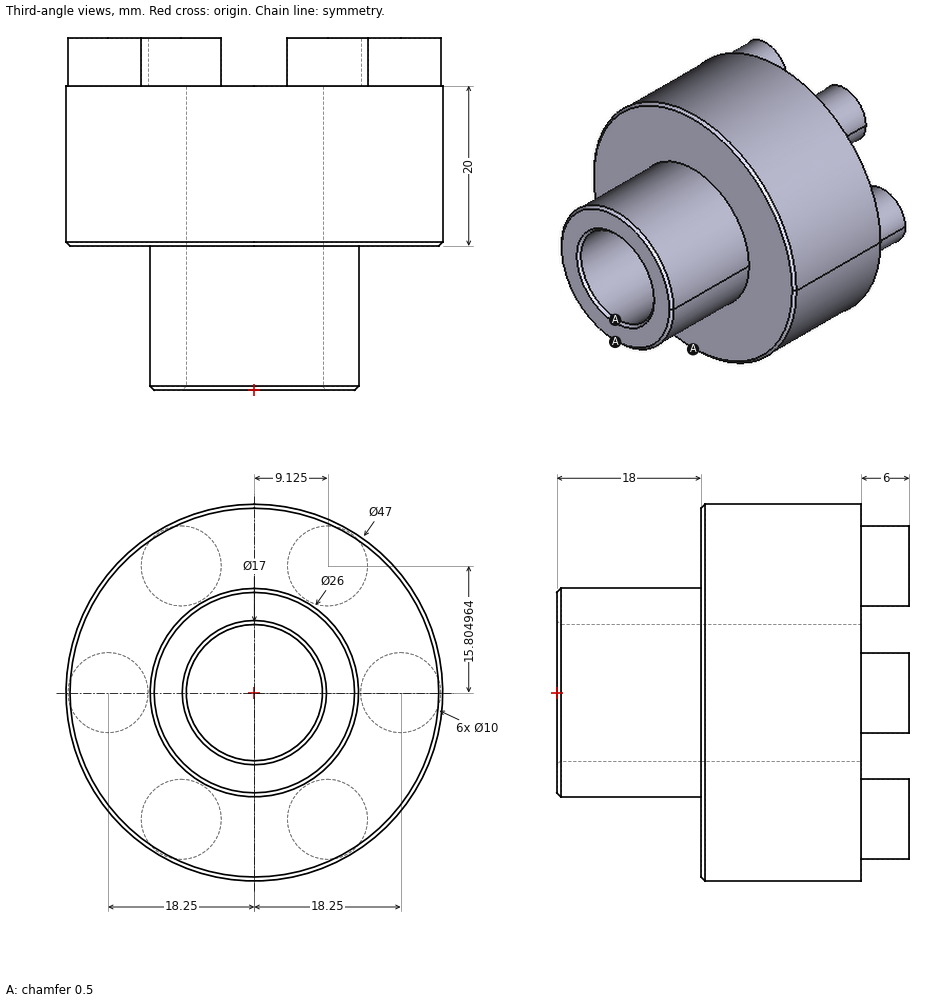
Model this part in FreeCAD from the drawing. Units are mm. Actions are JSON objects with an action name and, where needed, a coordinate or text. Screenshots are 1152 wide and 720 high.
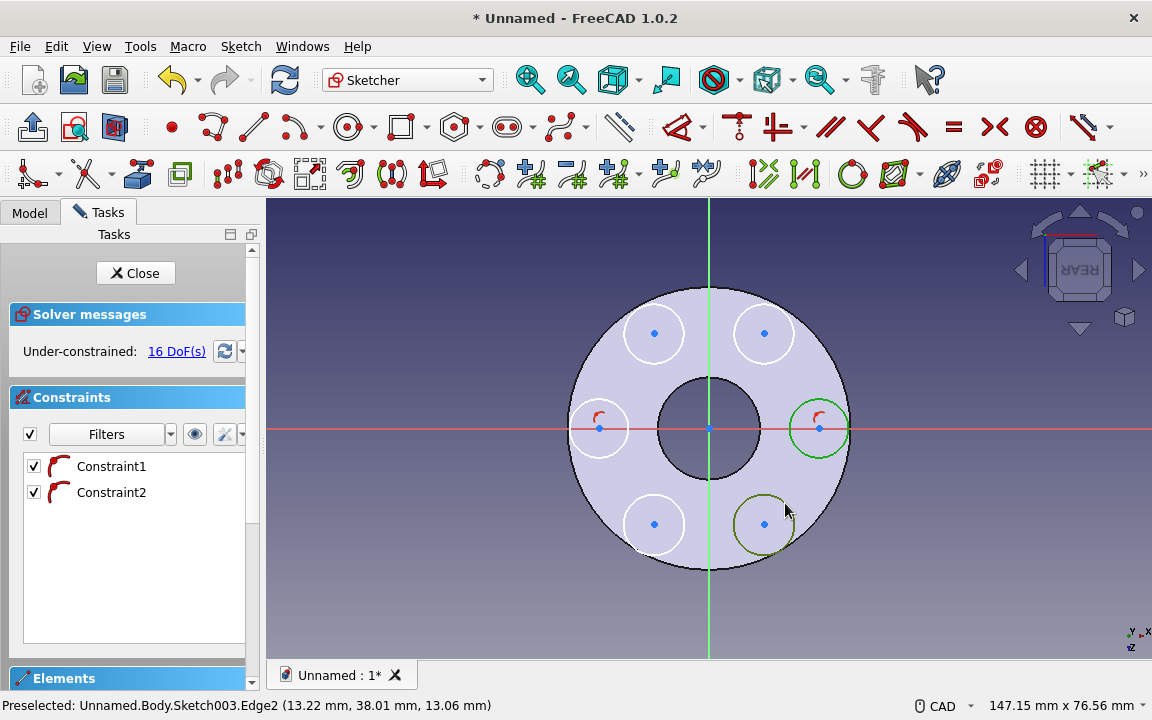
{"action": "left_click", "coordinate": [675, 503]}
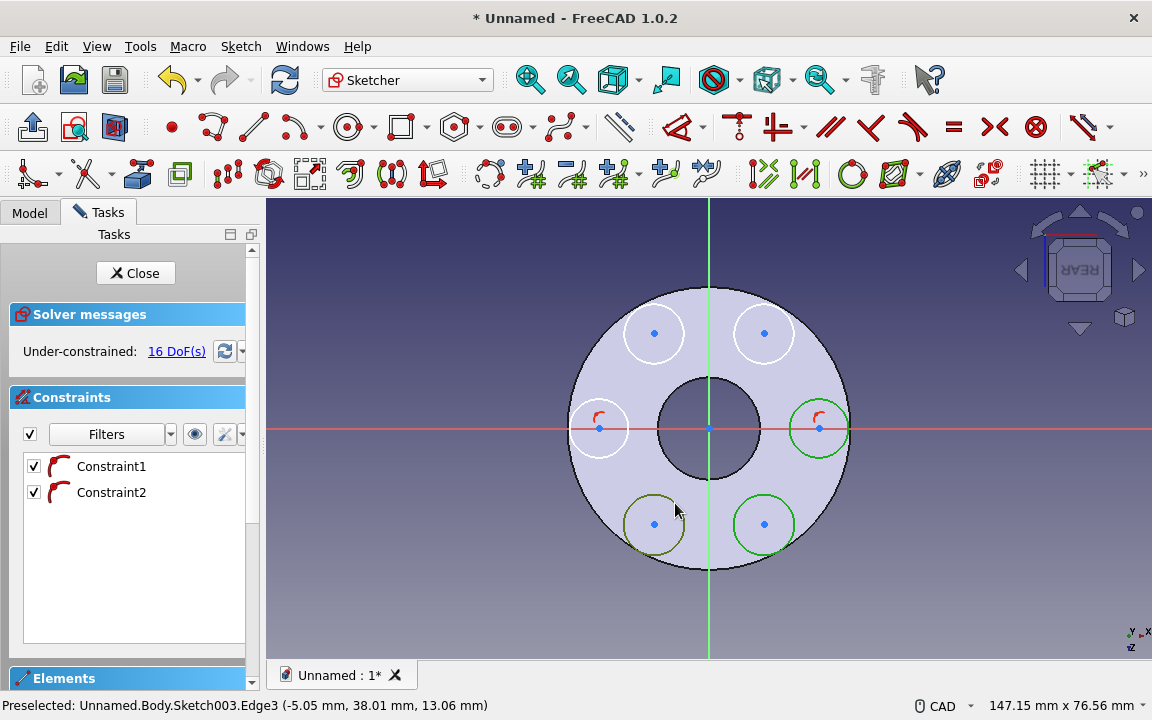
{"action": "left_click", "coordinate": [620, 408]}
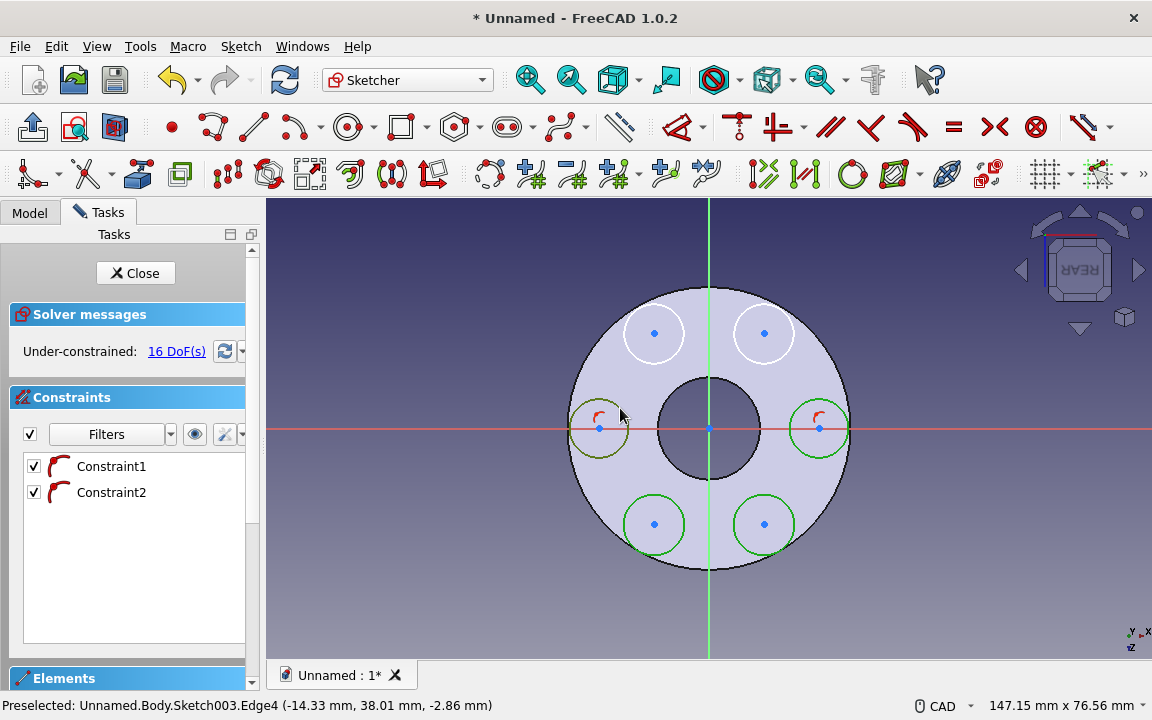
{"action": "left_click", "coordinate": [675, 313]}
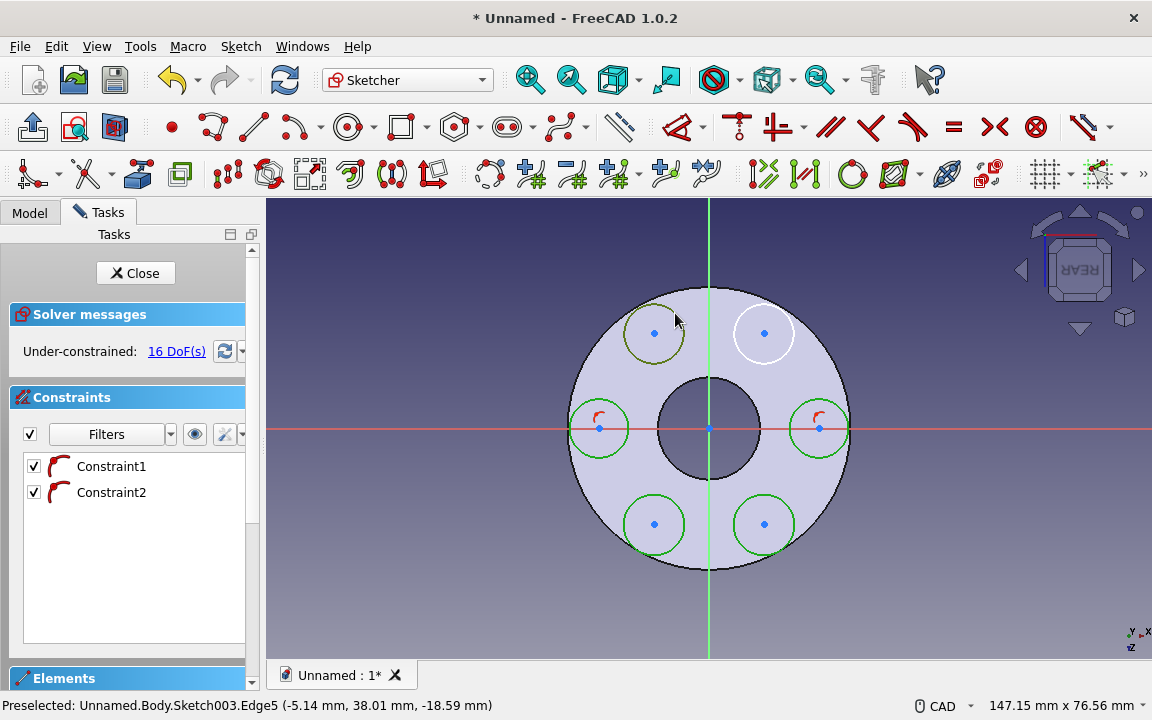
{"action": "left_click", "coordinate": [785, 313]}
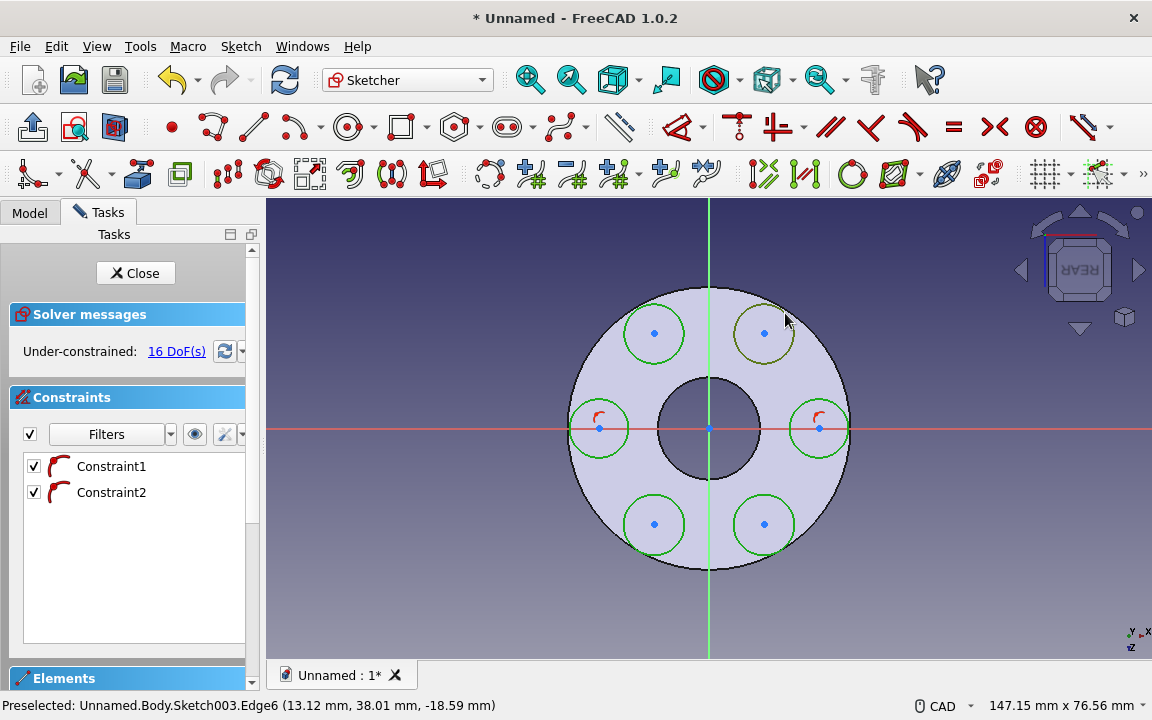
{"action": "left_click", "coordinate": [954, 128]}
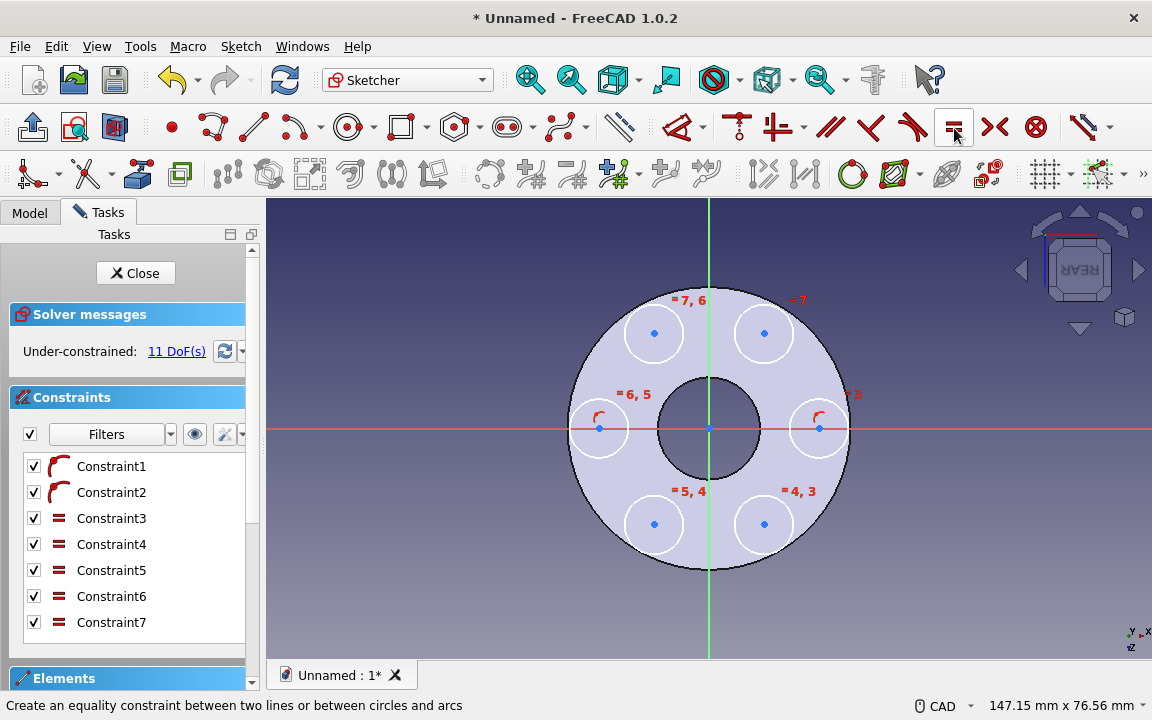
{"action": "left_click", "coordinate": [764, 525]}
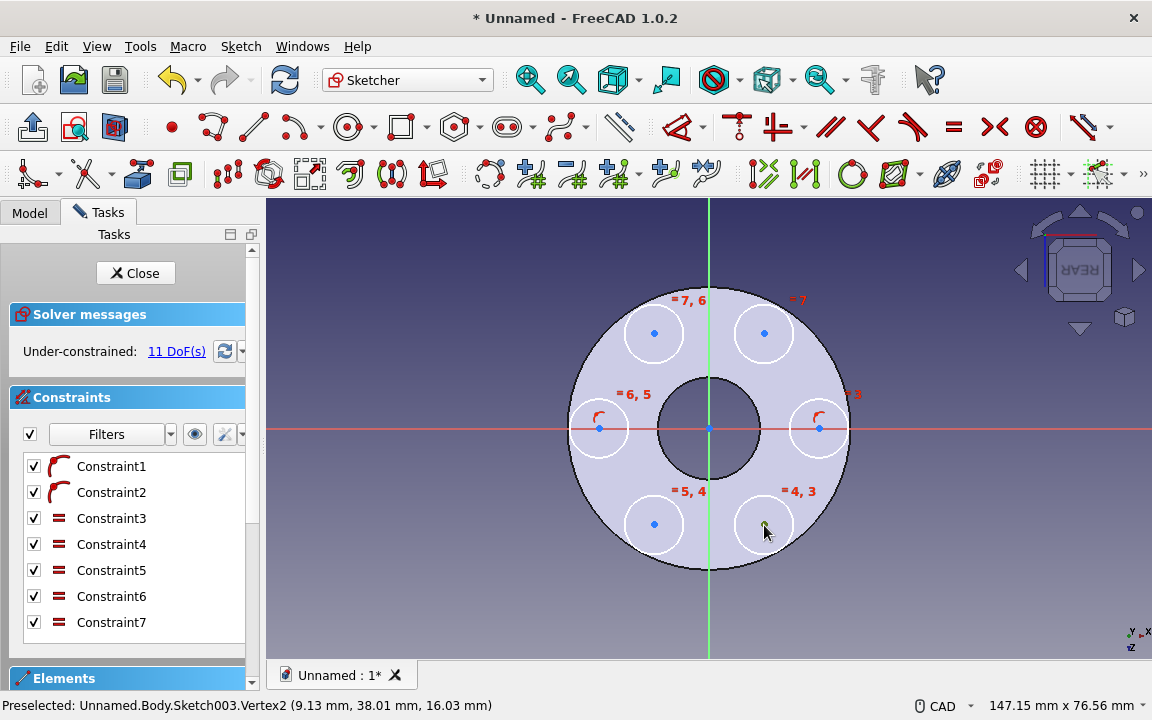
{"action": "left_click", "coordinate": [654, 525]}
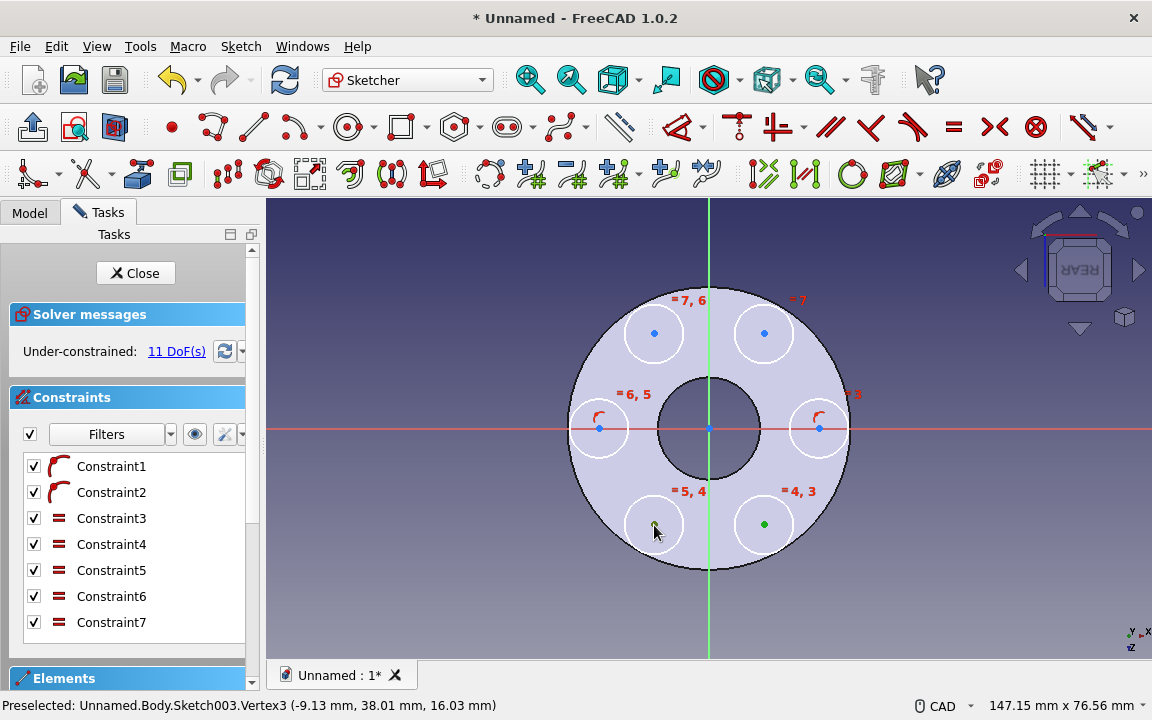
{"action": "left_click", "coordinate": [709, 602]}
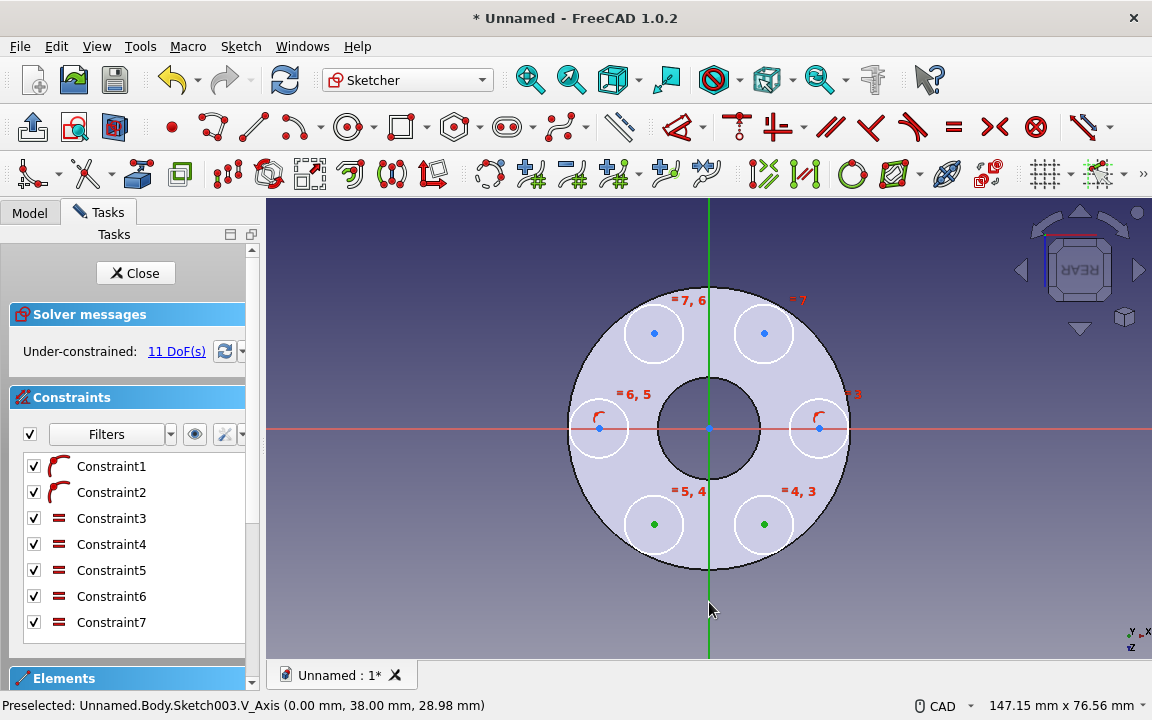
{"action": "left_click", "coordinate": [995, 128]}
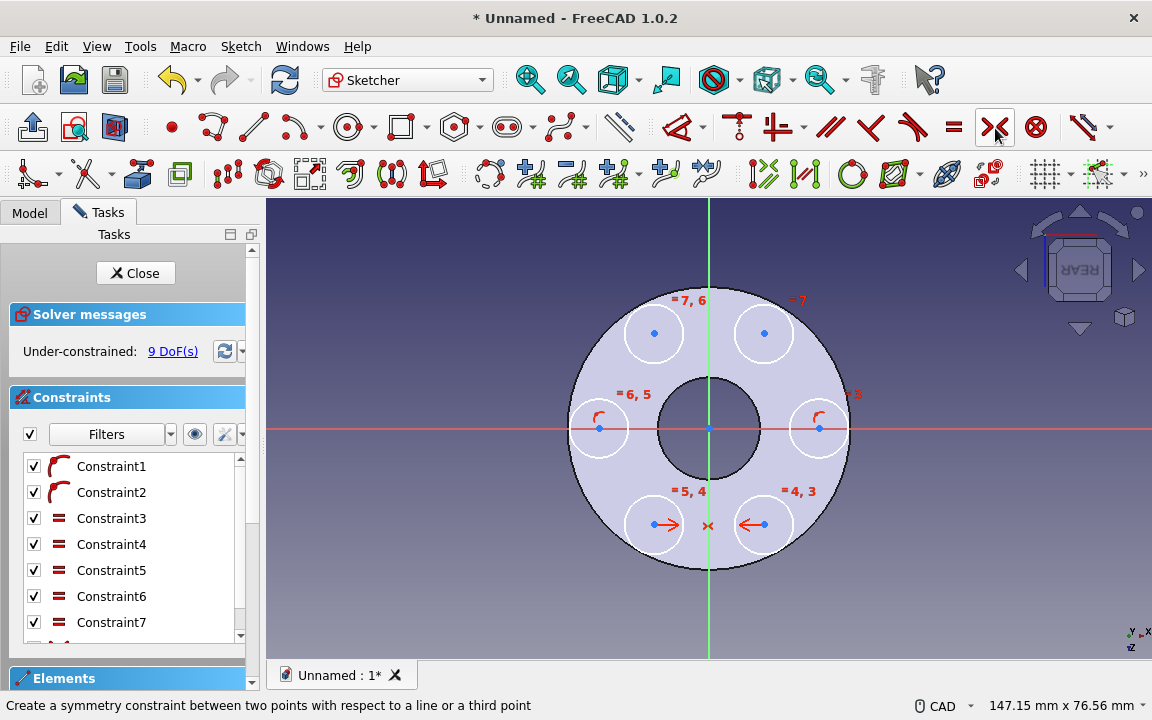
{"action": "left_click", "coordinate": [654, 525]}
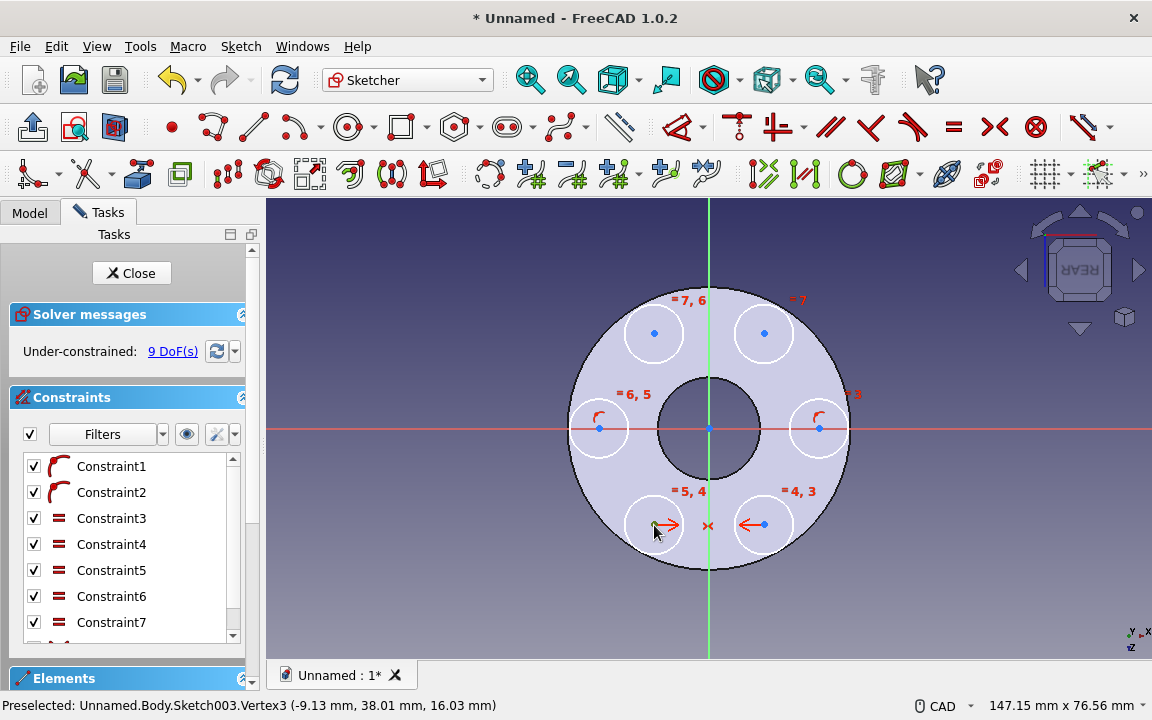
{"action": "left_click", "coordinate": [654, 334]}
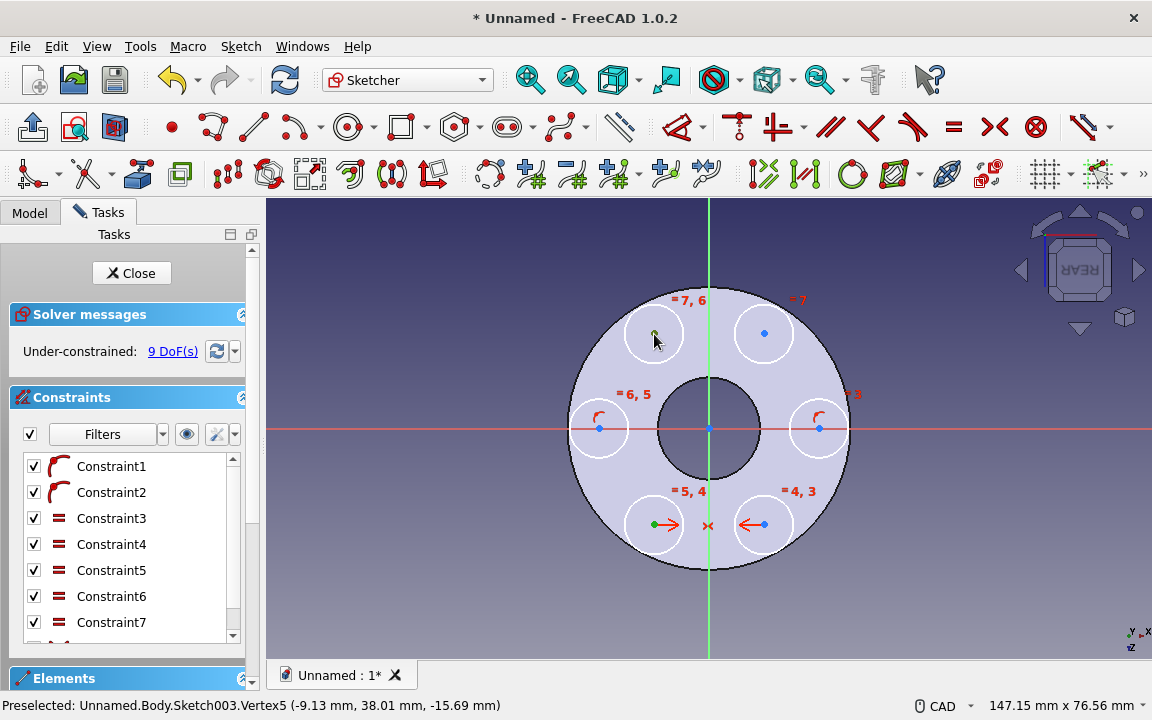
{"action": "left_click", "coordinate": [344, 429]}